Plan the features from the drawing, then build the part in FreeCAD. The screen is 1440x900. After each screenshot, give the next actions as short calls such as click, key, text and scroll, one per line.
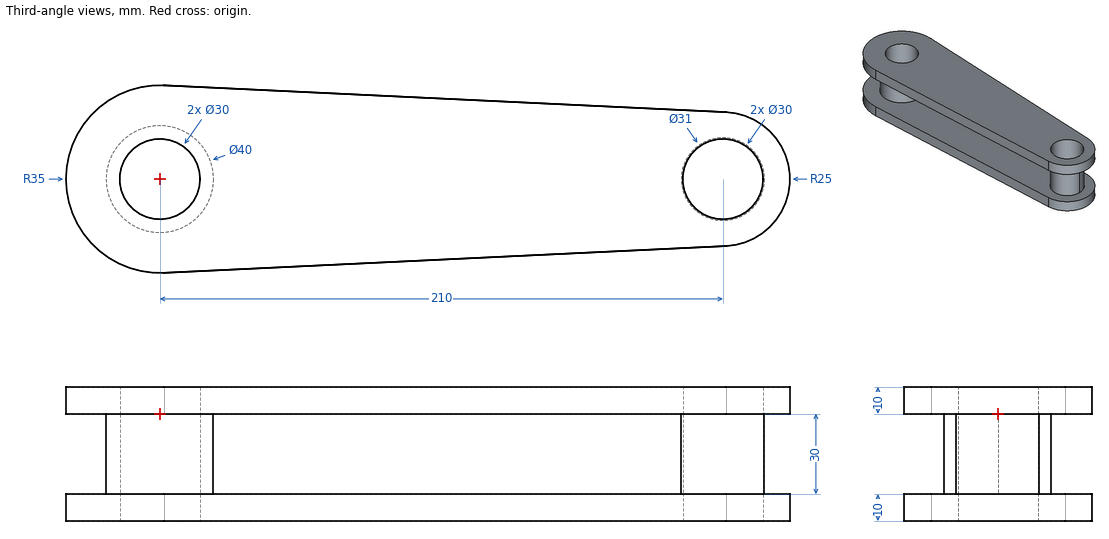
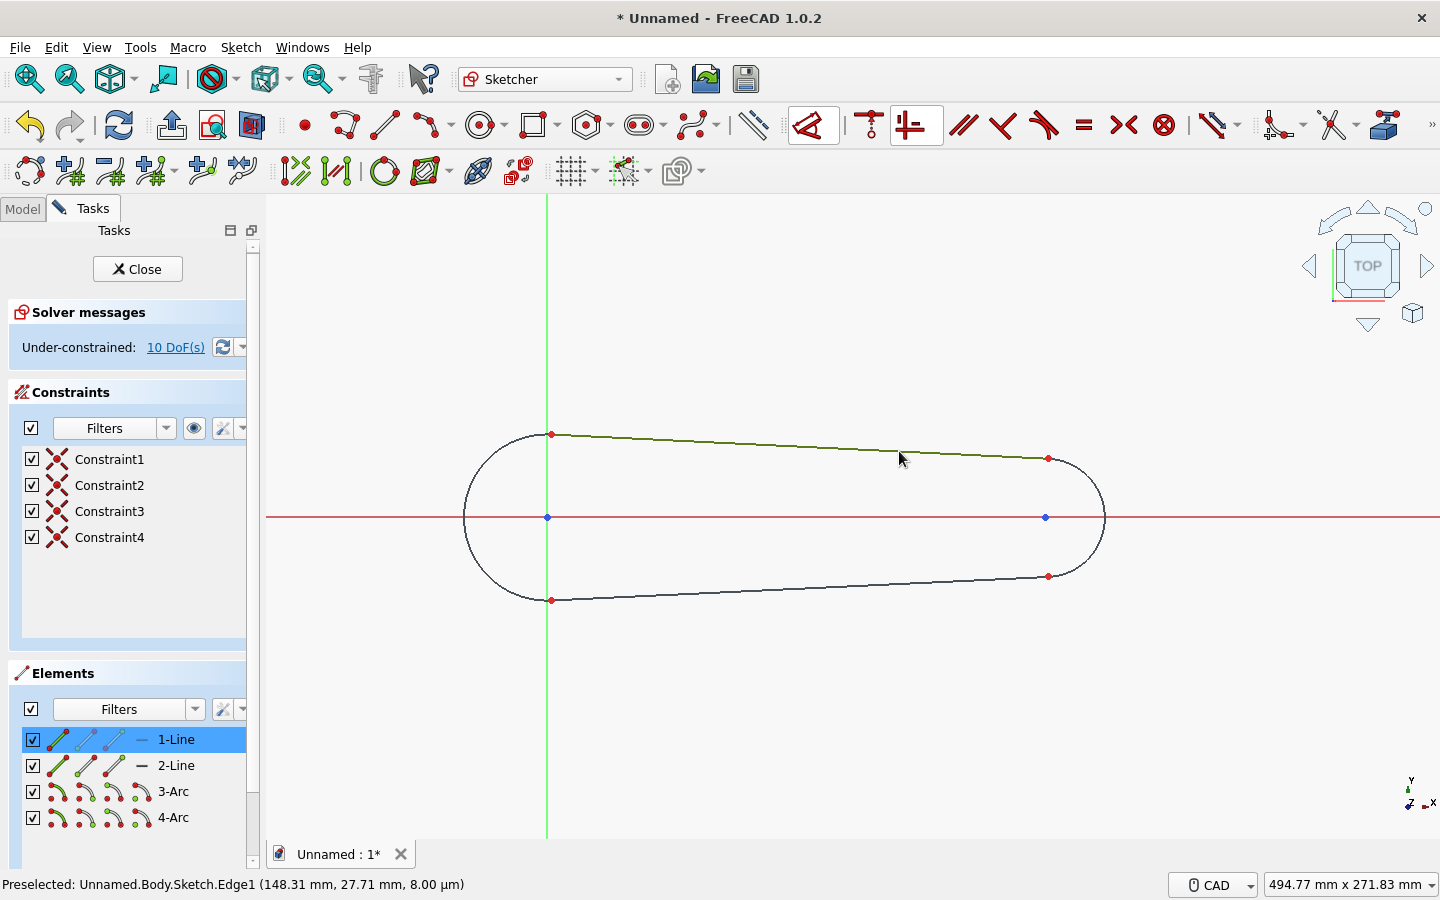
click(481, 467)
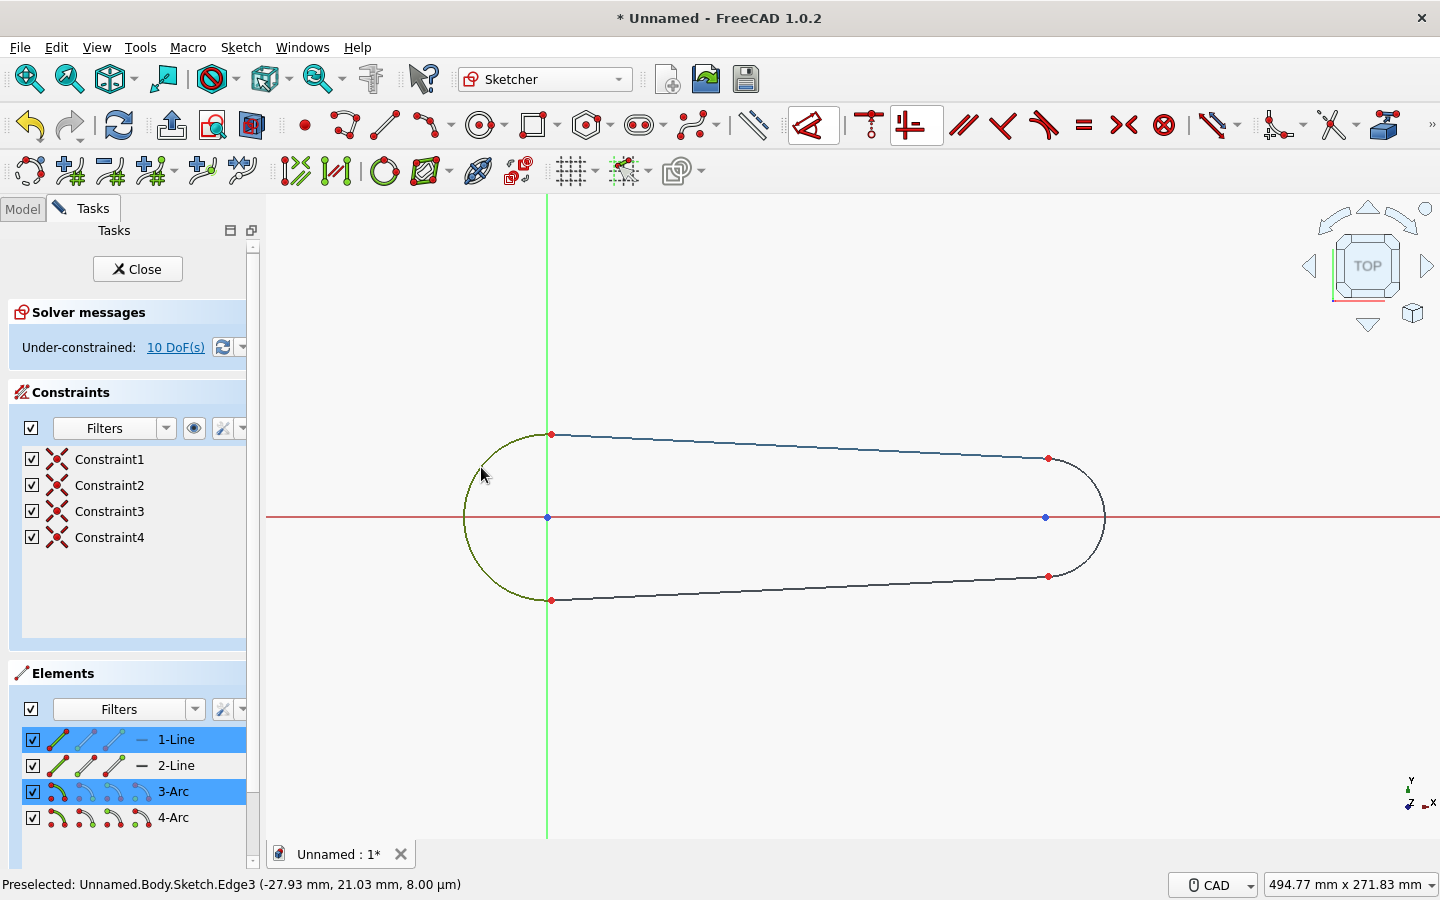
click(1044, 126)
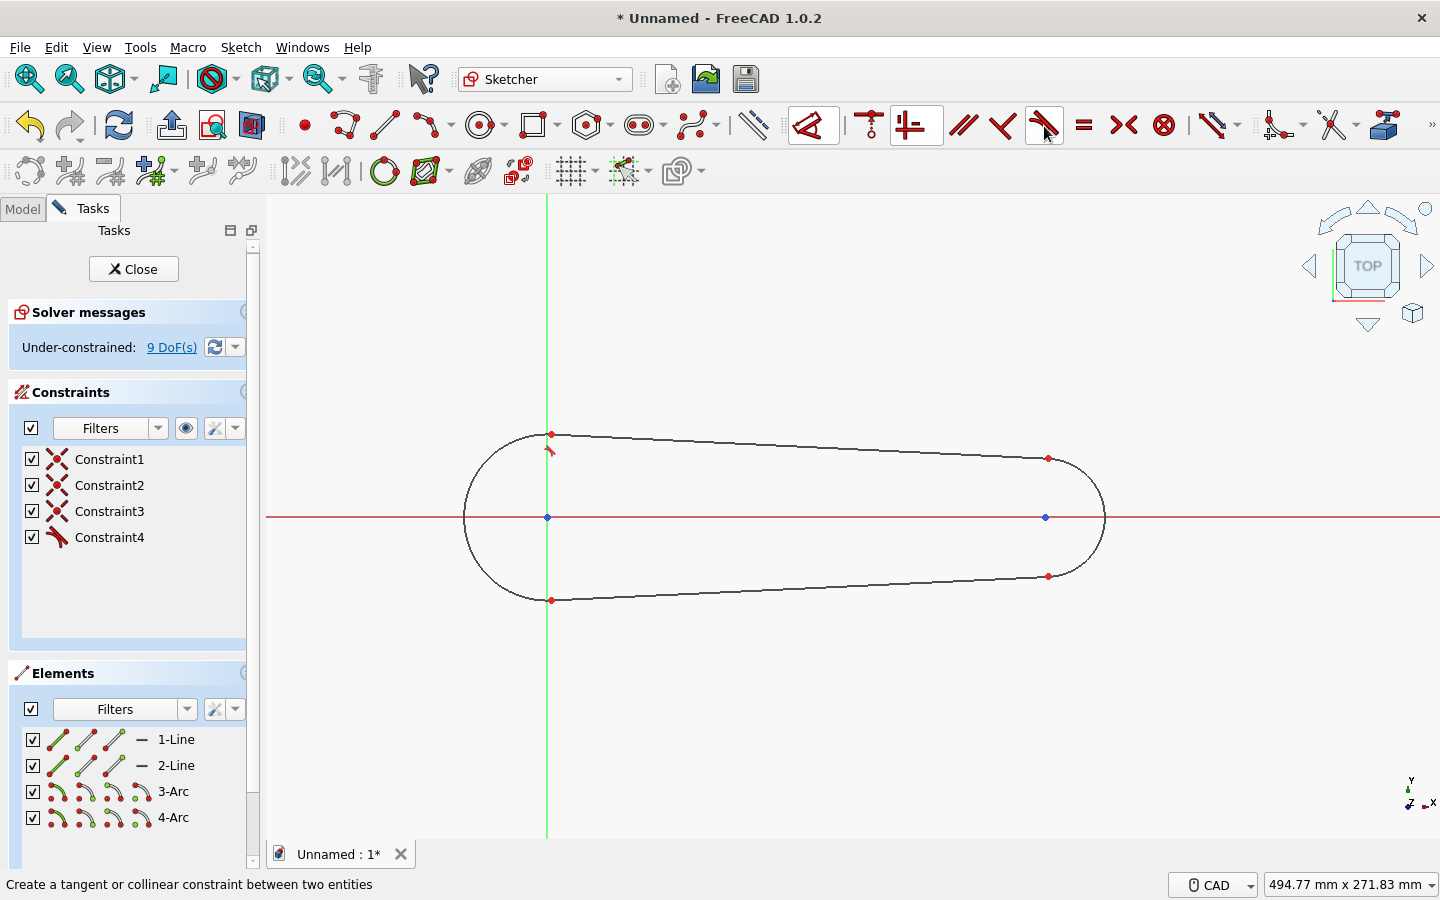
click(899, 451)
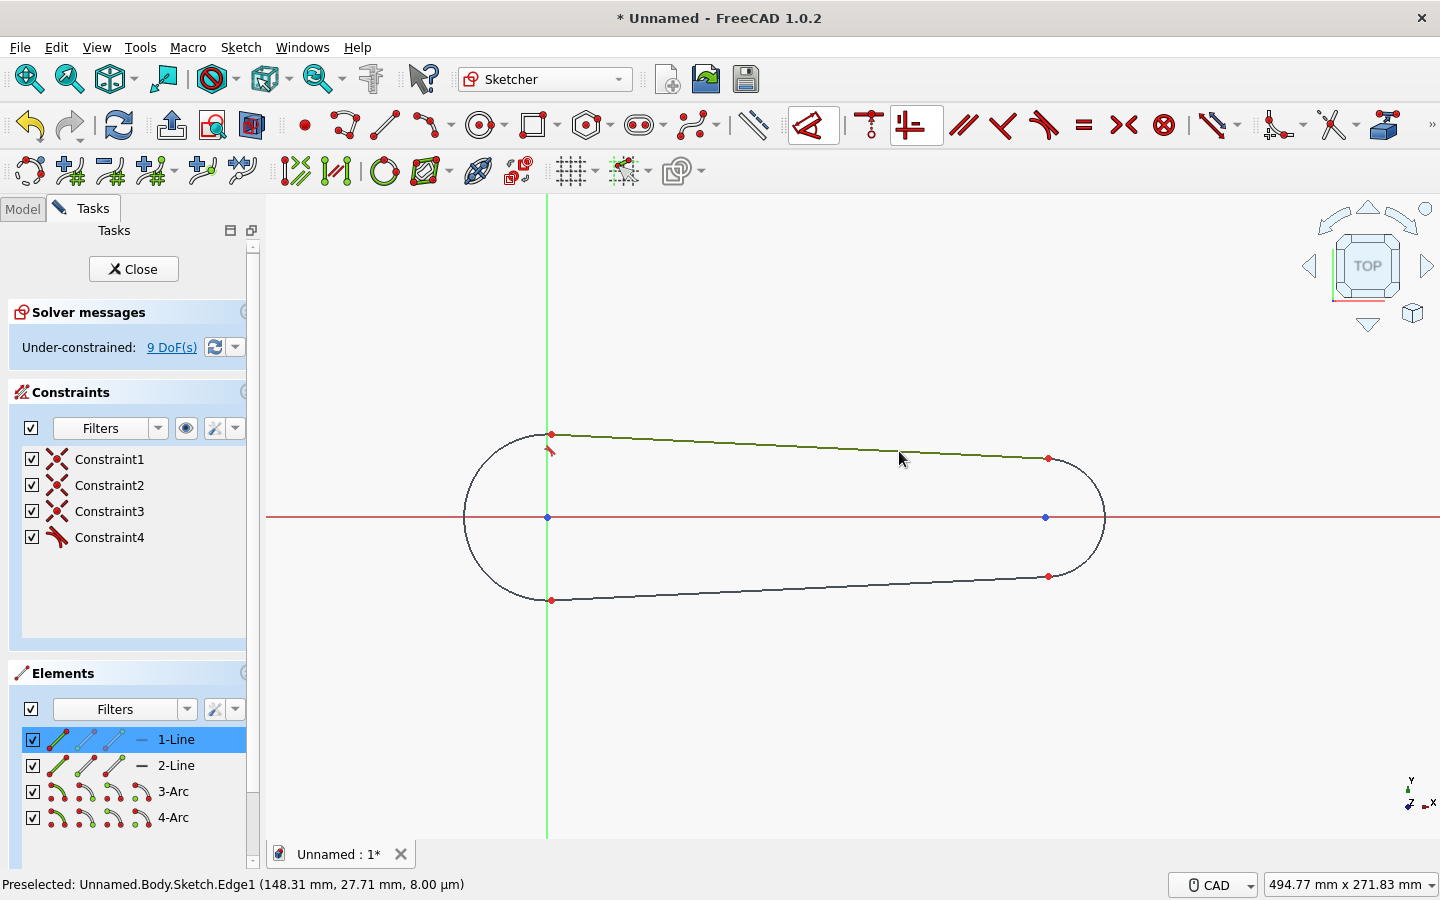
click(1094, 552)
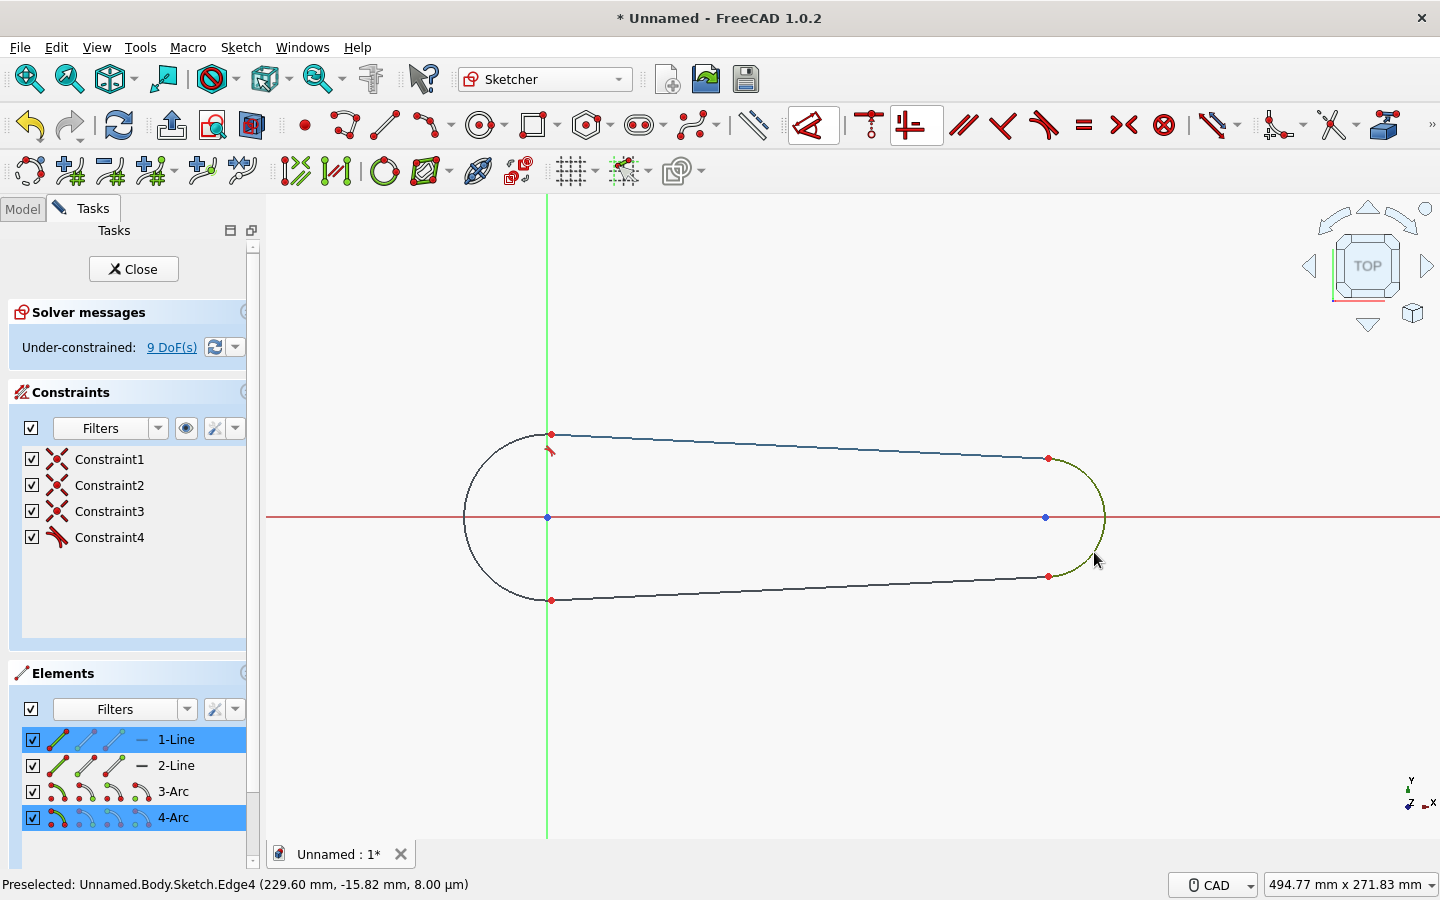
key(t)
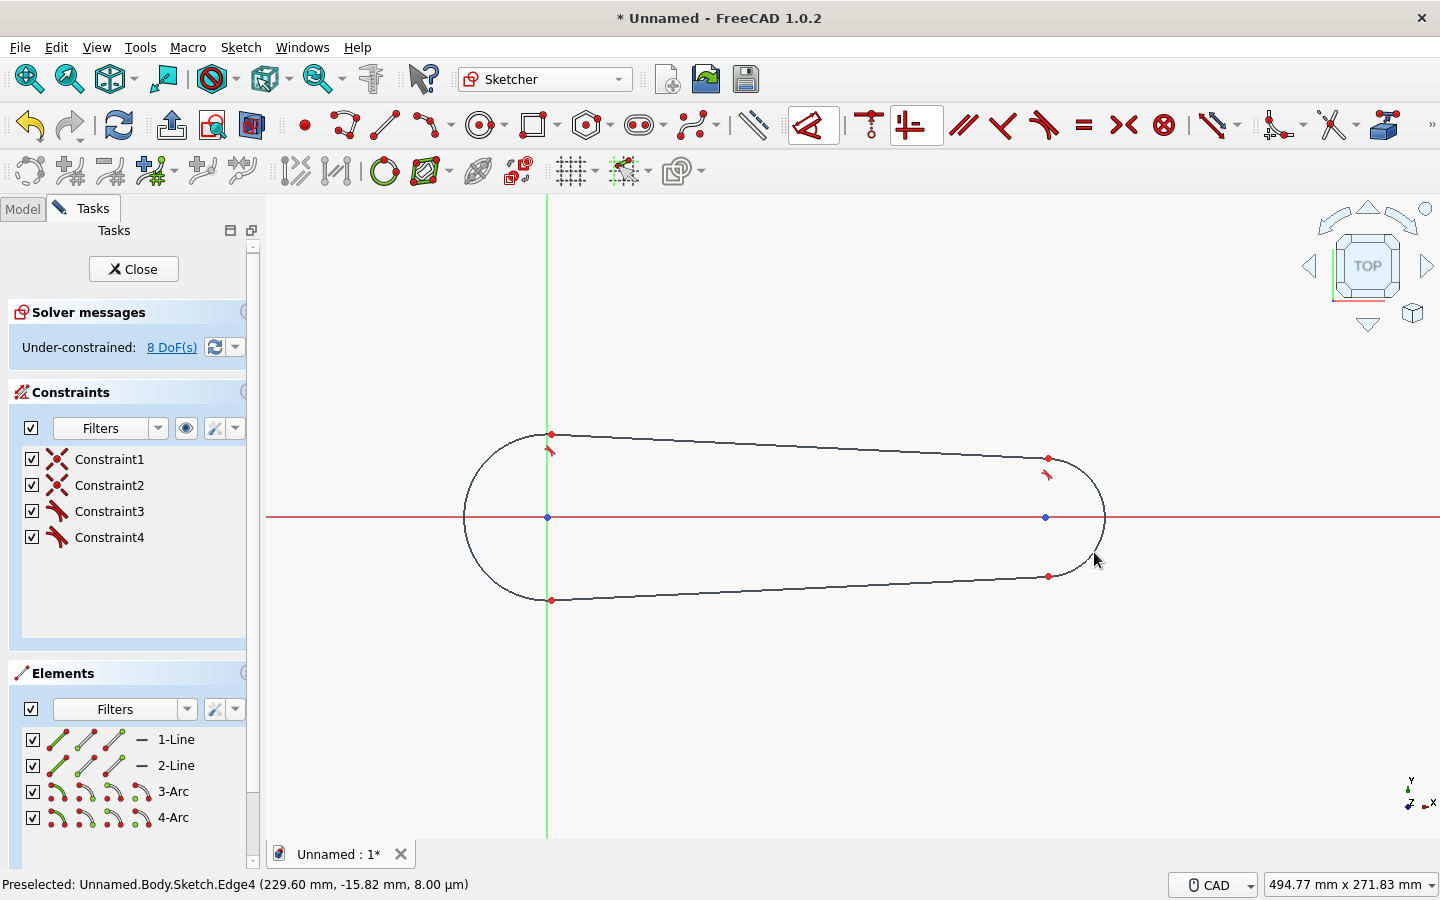
click(700, 593)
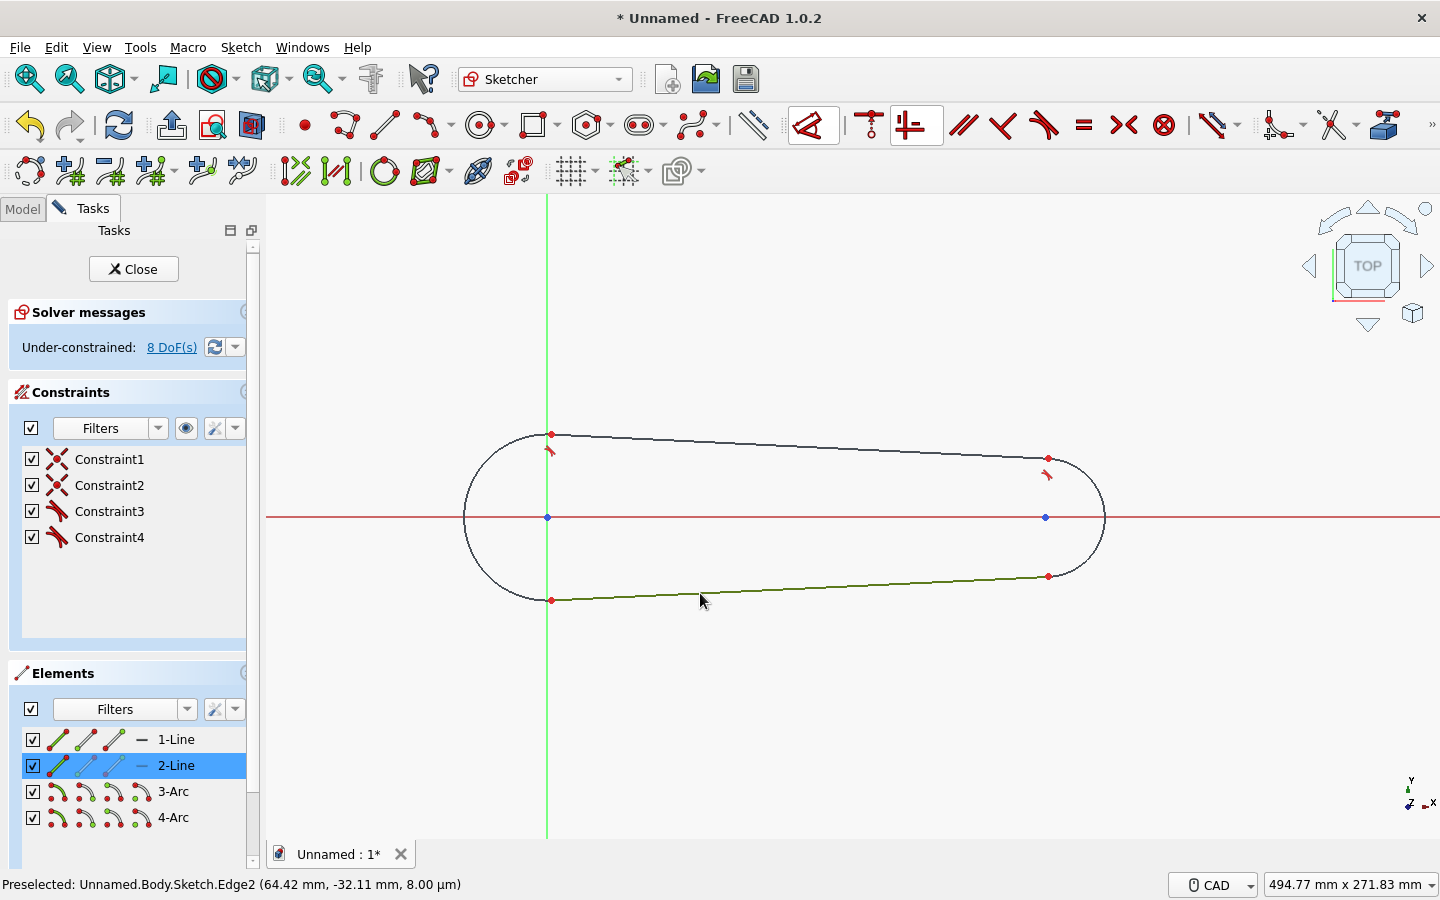
click(481, 467)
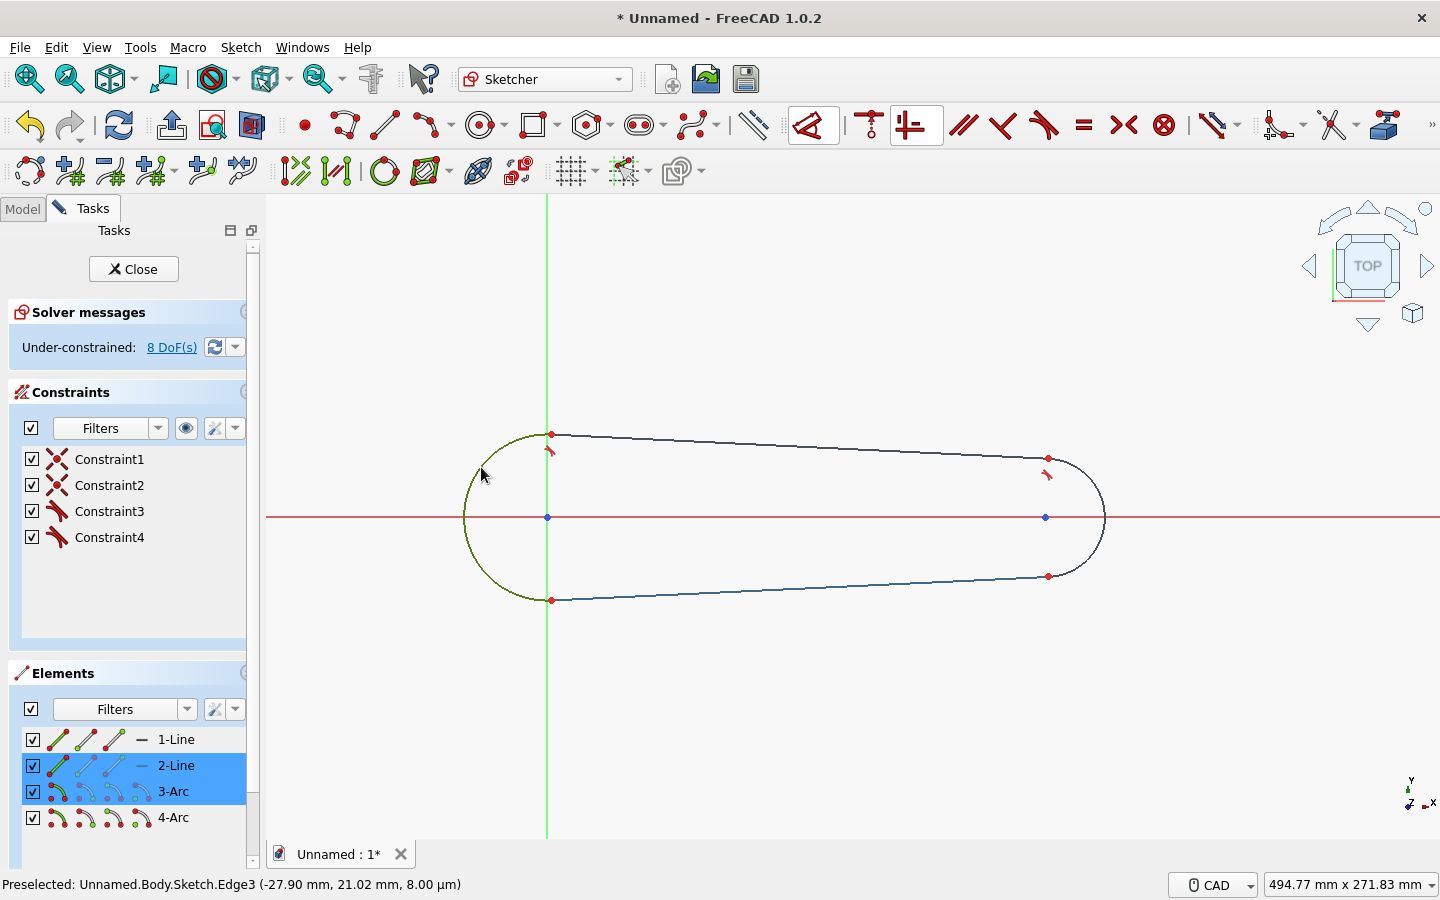
key(t)